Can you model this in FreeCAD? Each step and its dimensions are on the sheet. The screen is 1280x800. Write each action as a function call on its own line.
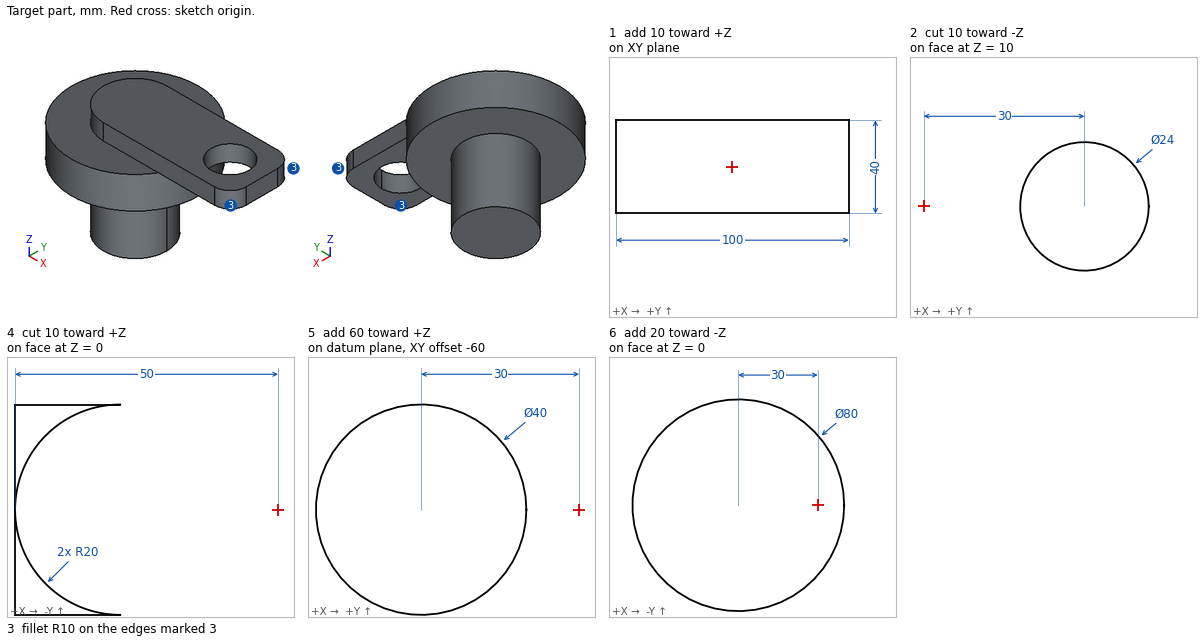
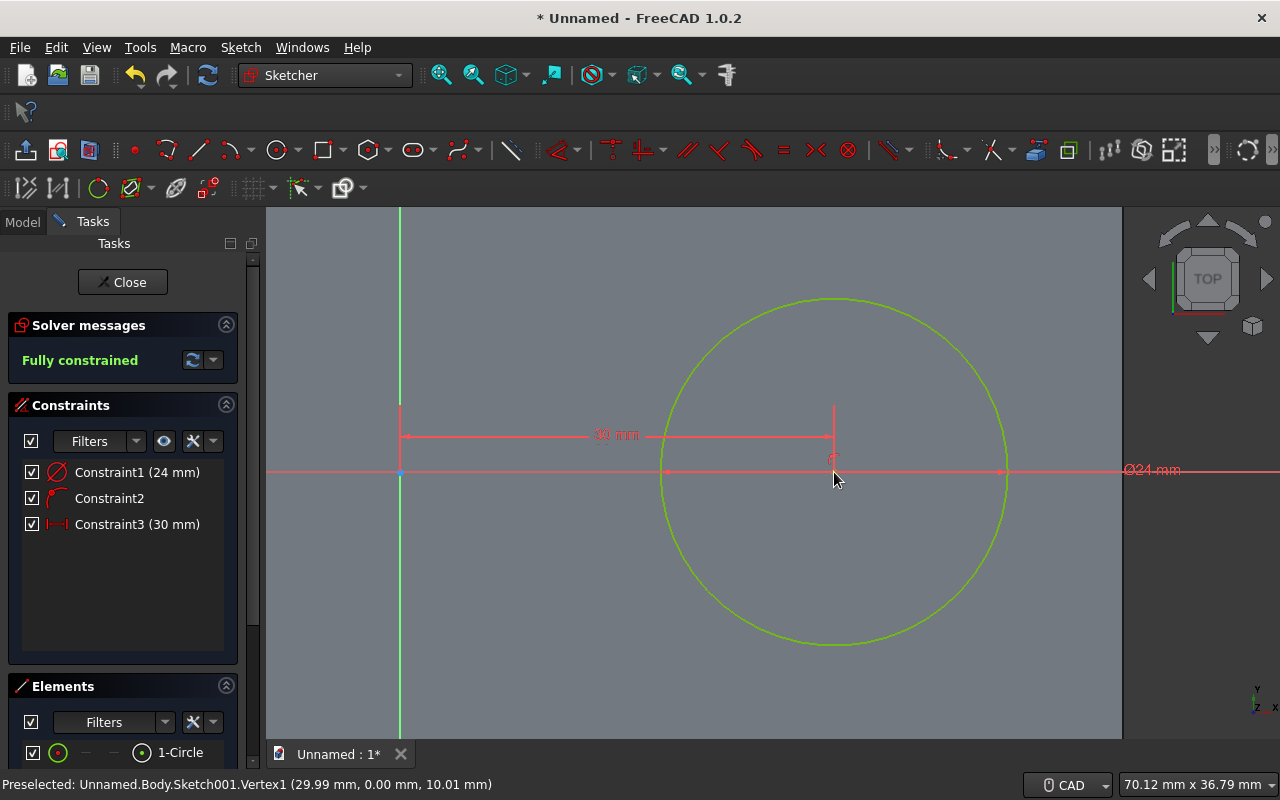
click(123, 282)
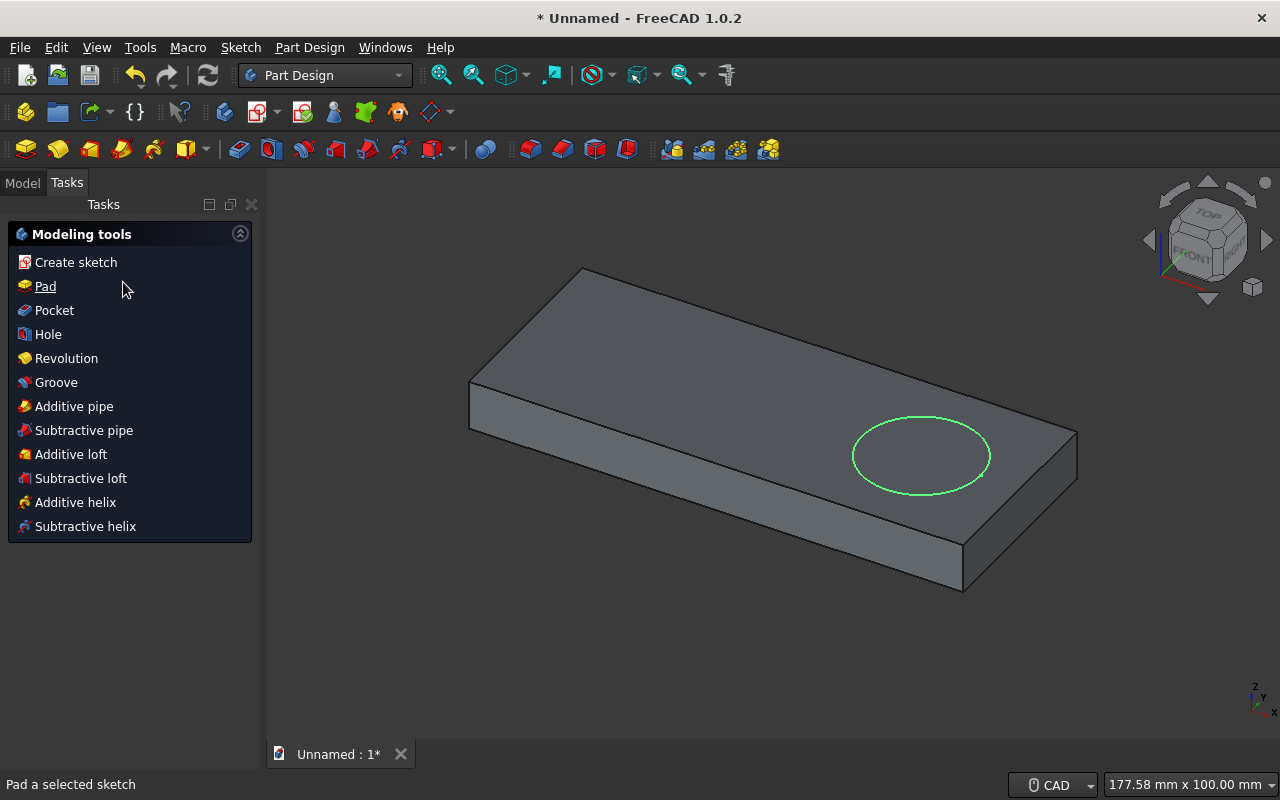
click(240, 150)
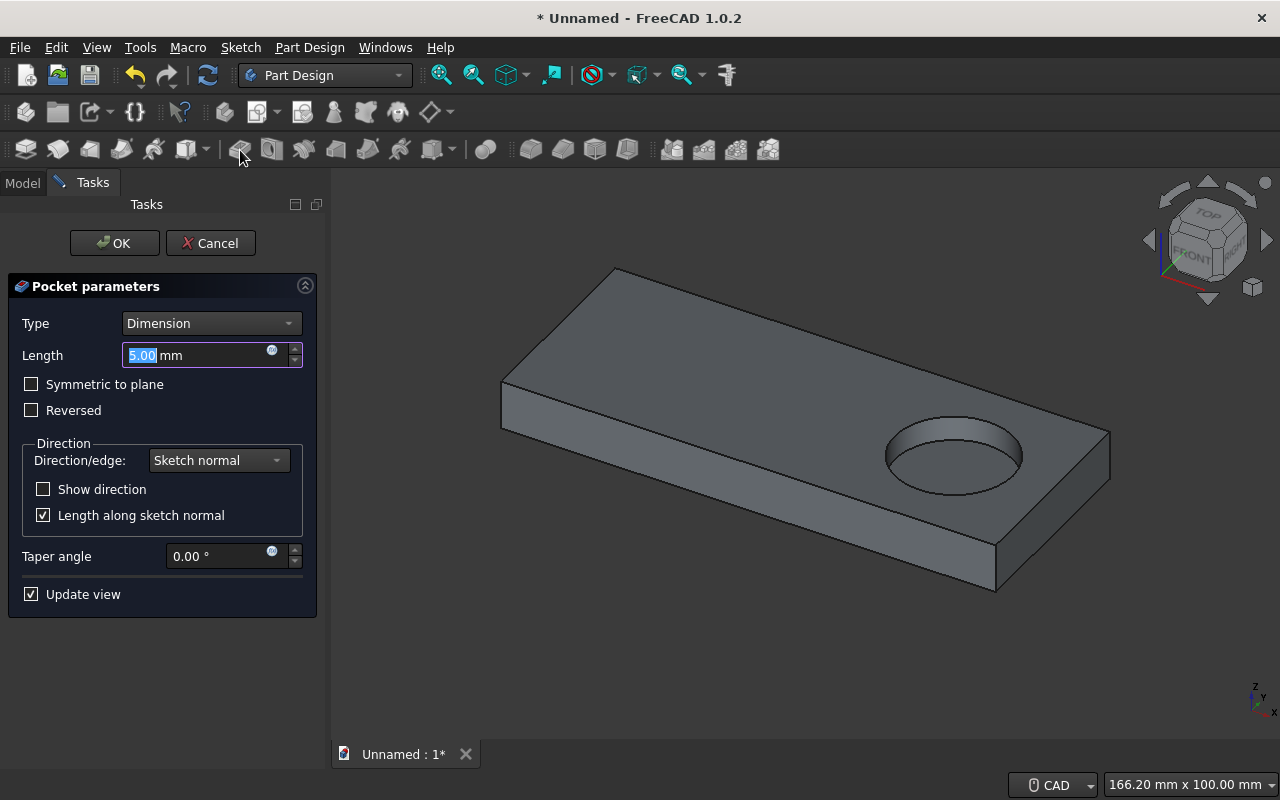
text(10)
key(Tab)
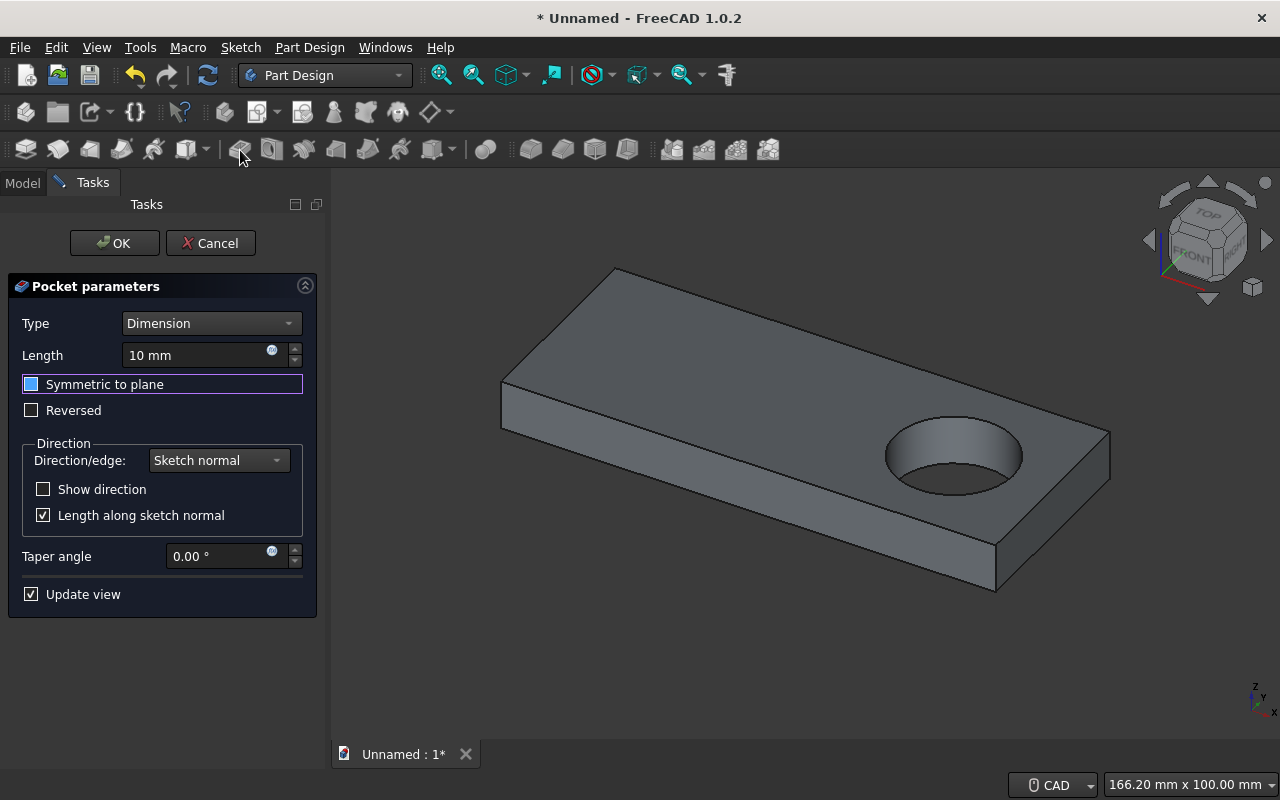
click(115, 243)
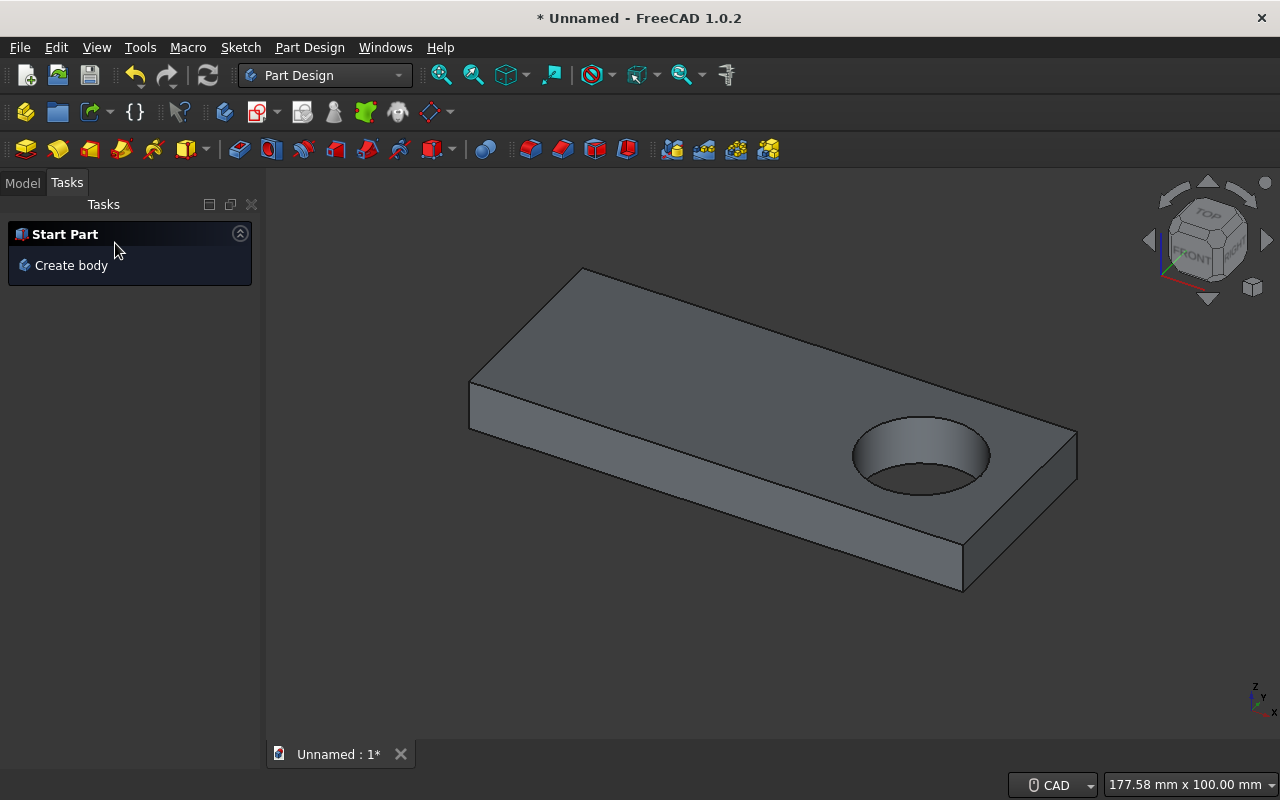
click(963, 568)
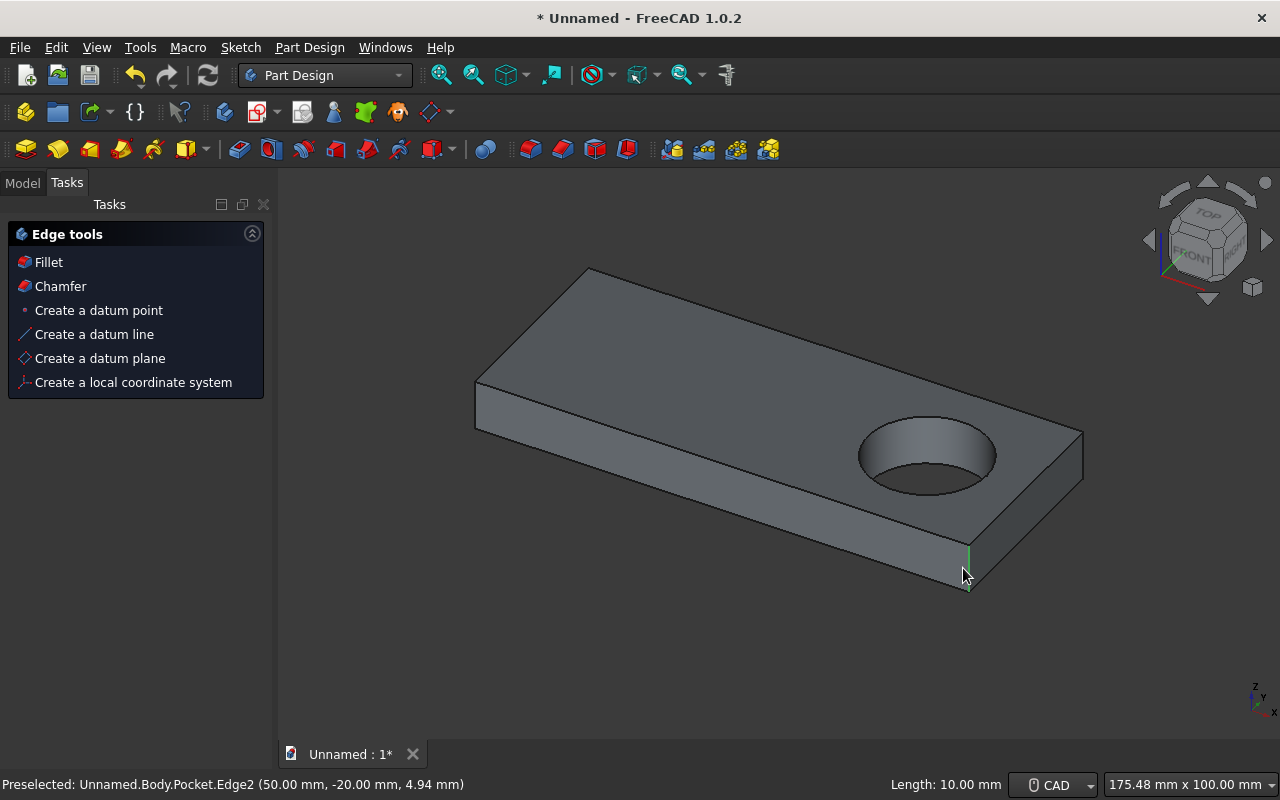
key(0)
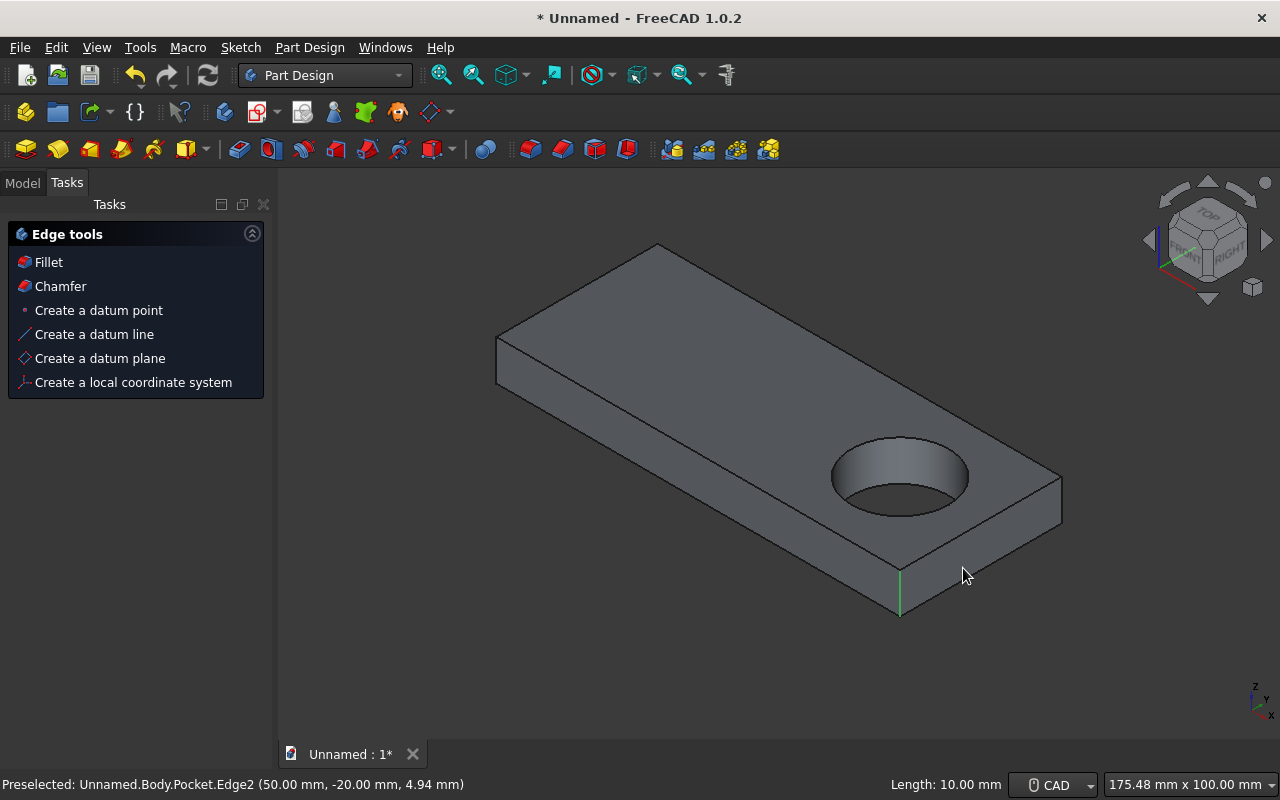
key(2)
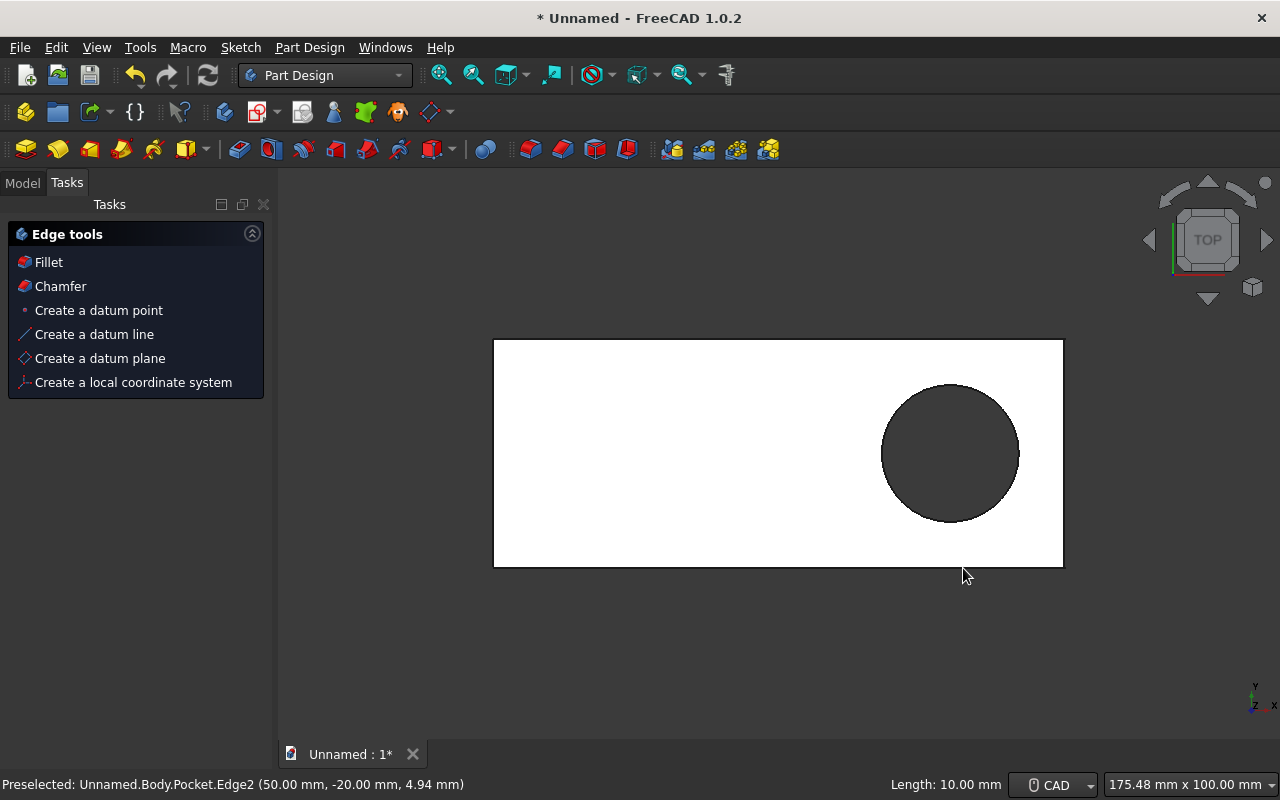
key(1)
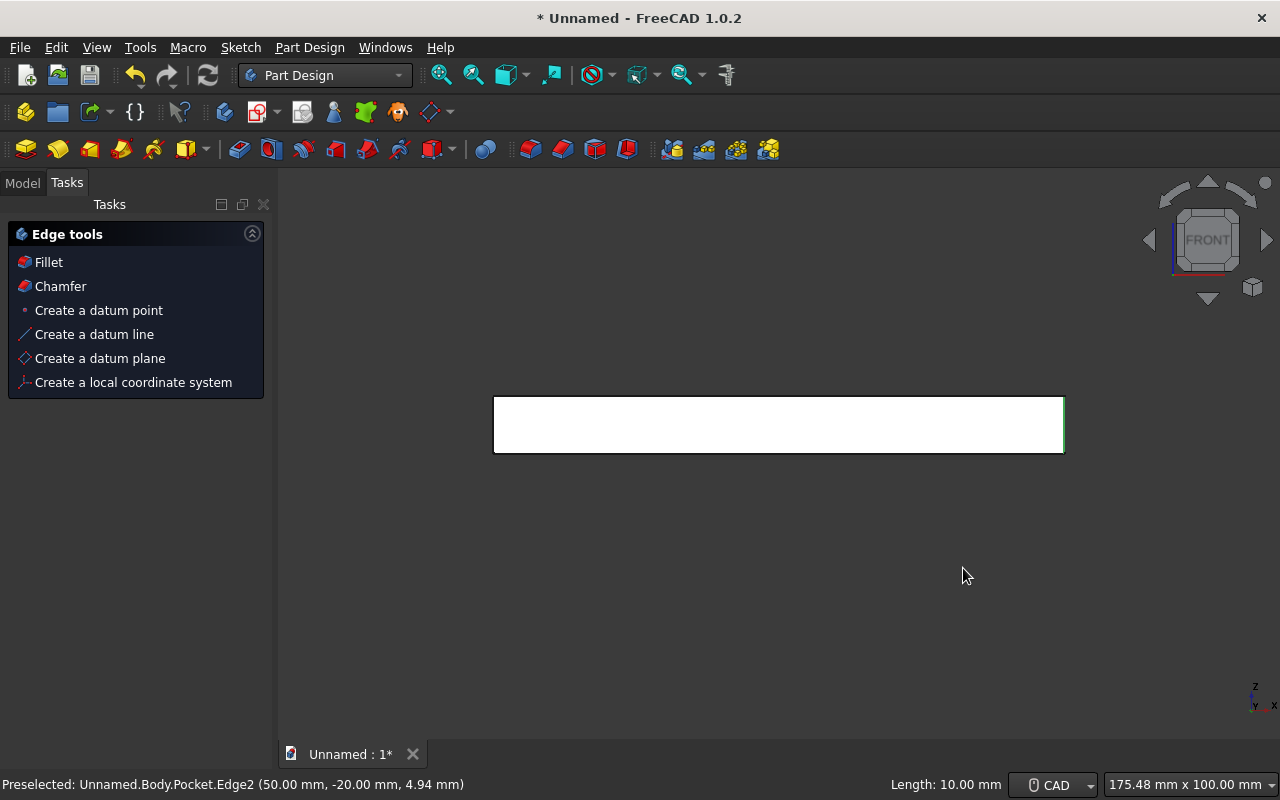
key(3)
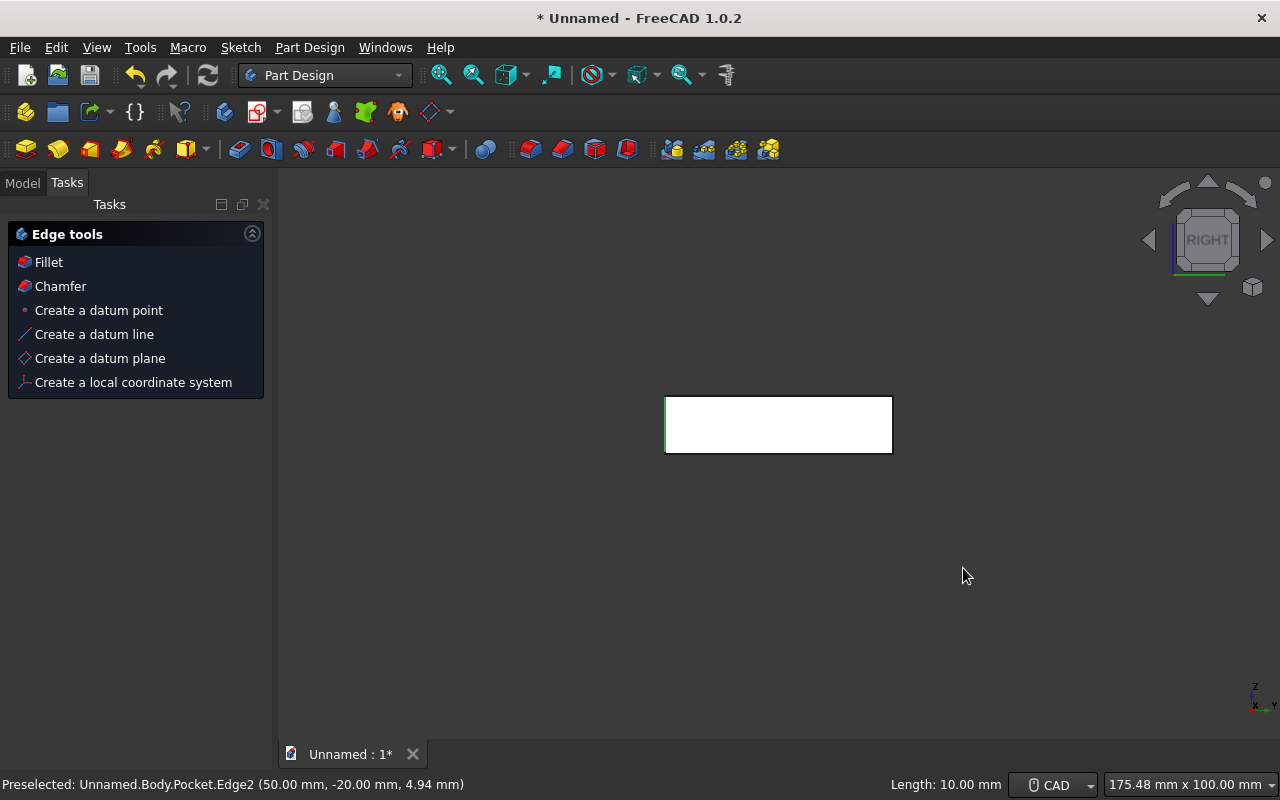
click(442, 76)